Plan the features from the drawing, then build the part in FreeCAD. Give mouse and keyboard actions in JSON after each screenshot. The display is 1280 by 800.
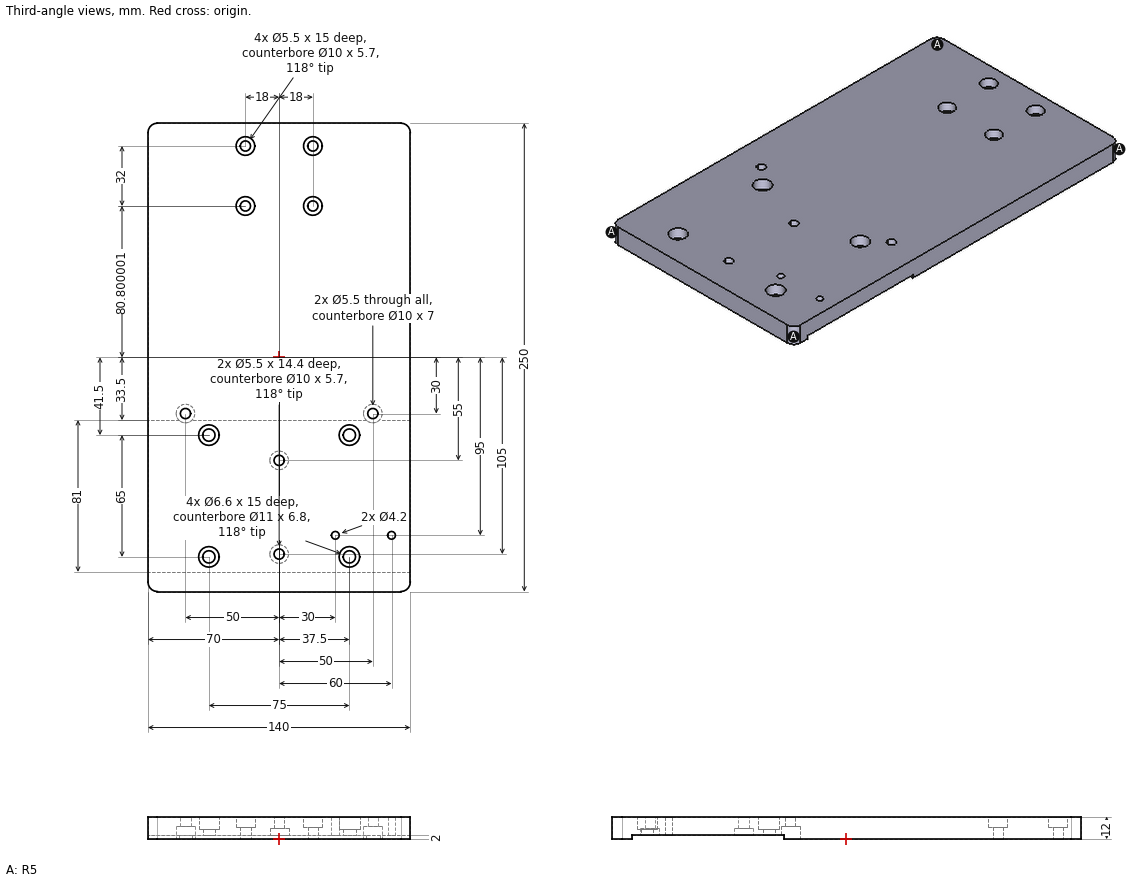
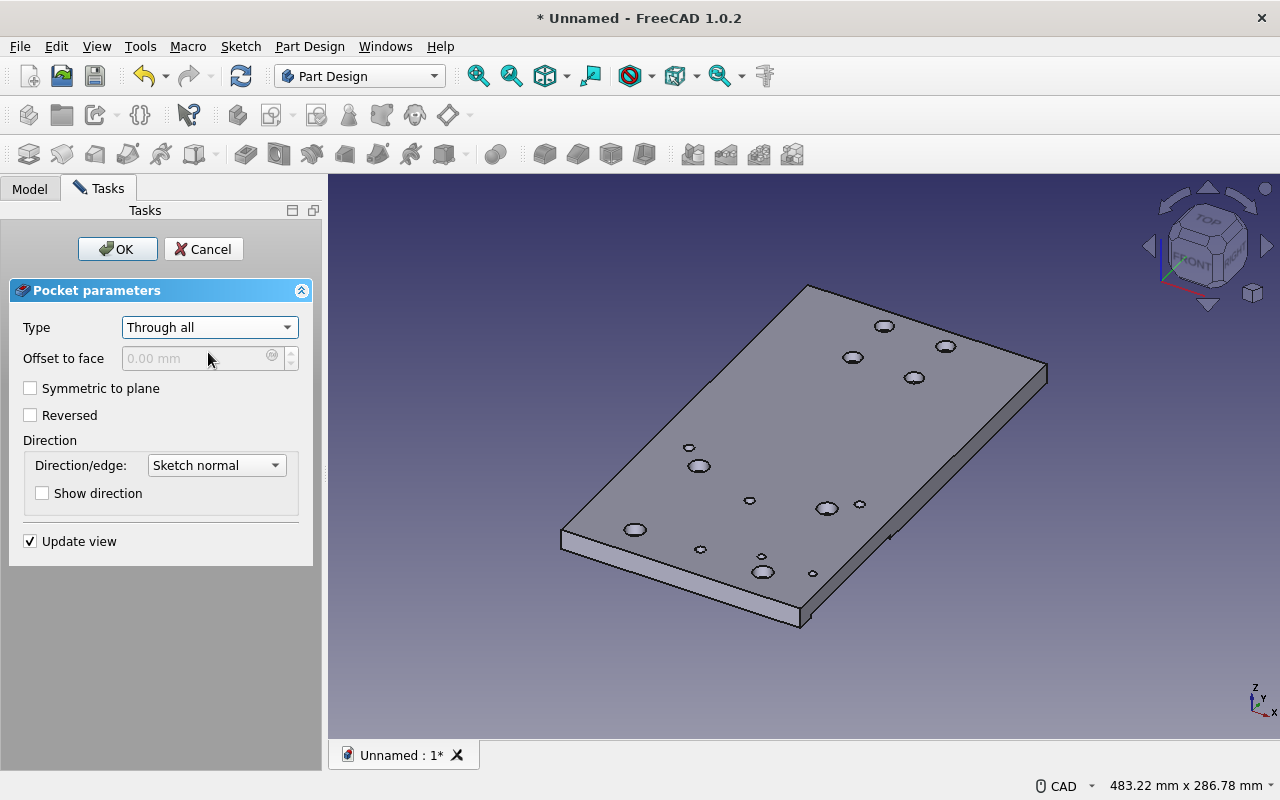
{"action": "left_click", "coordinate": [118, 249]}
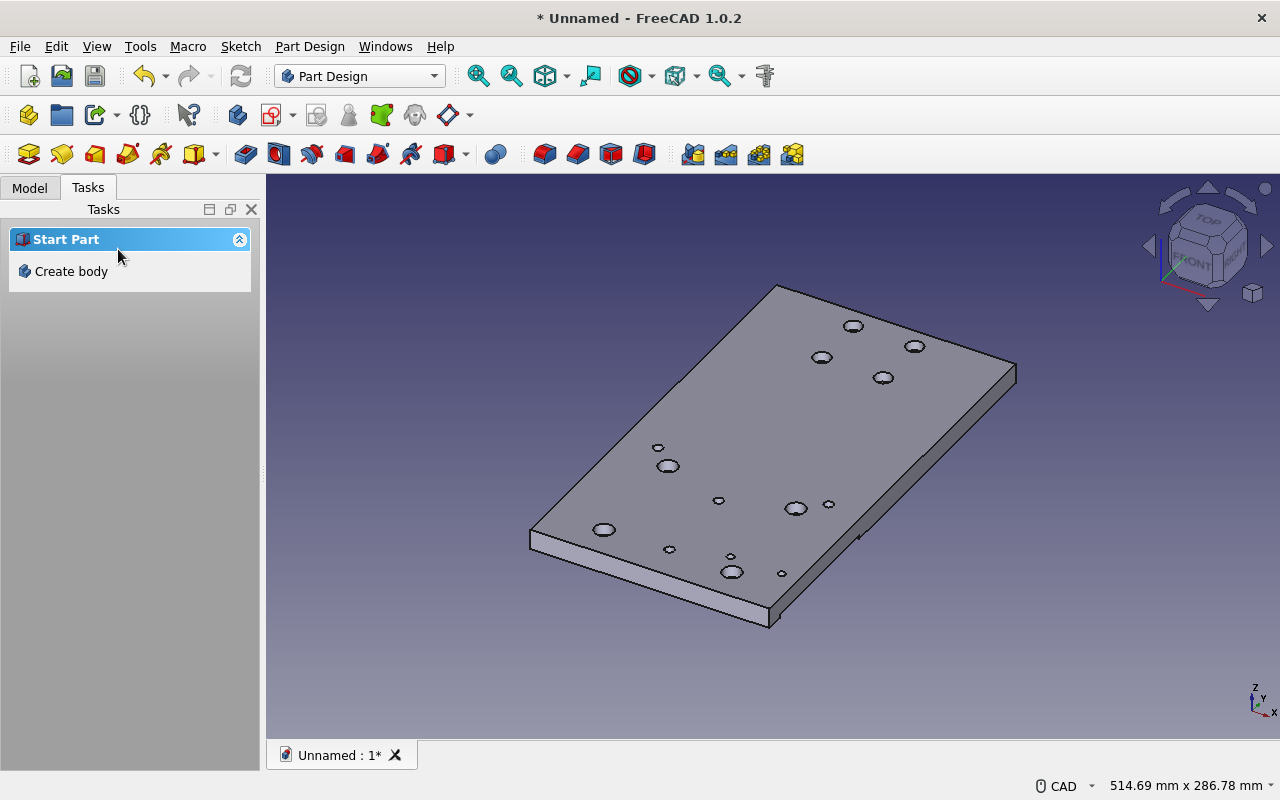
{"action": "left_click", "coordinate": [769, 617]}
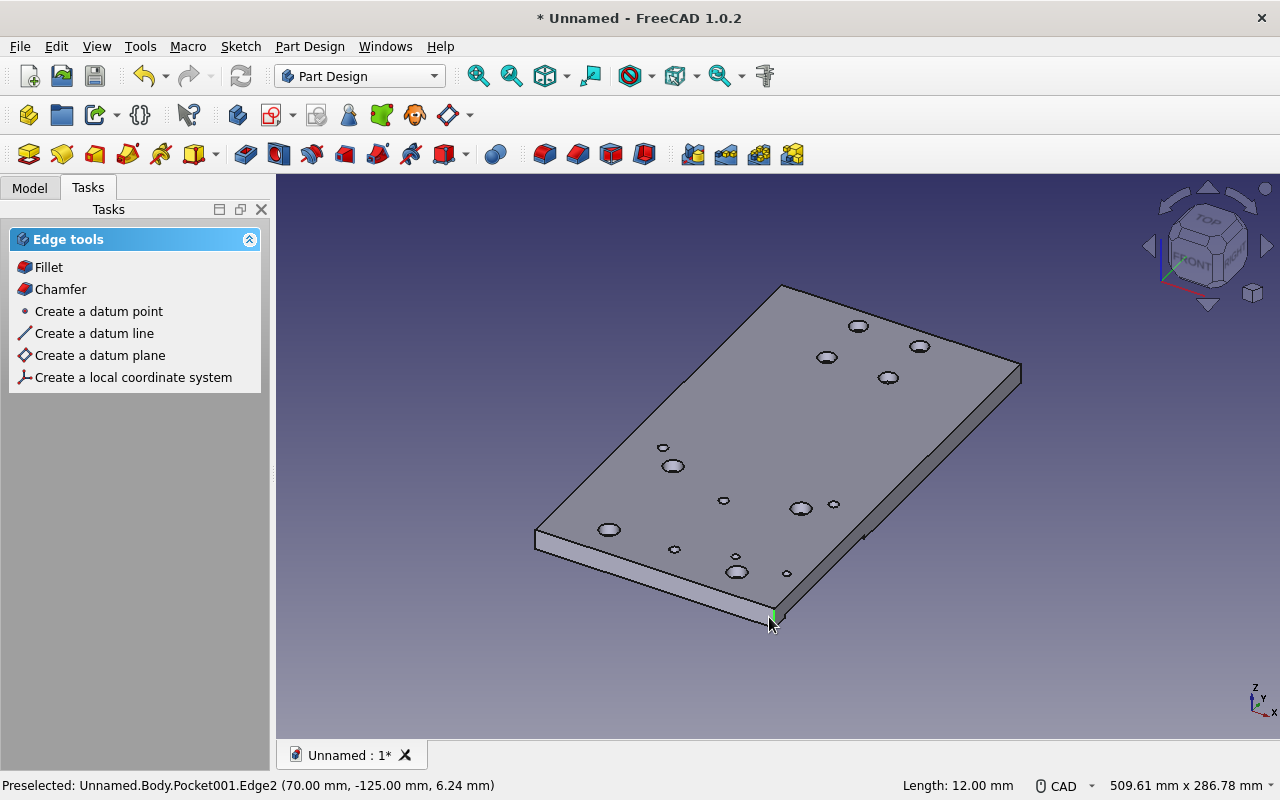
{"action": "key", "text": "0"}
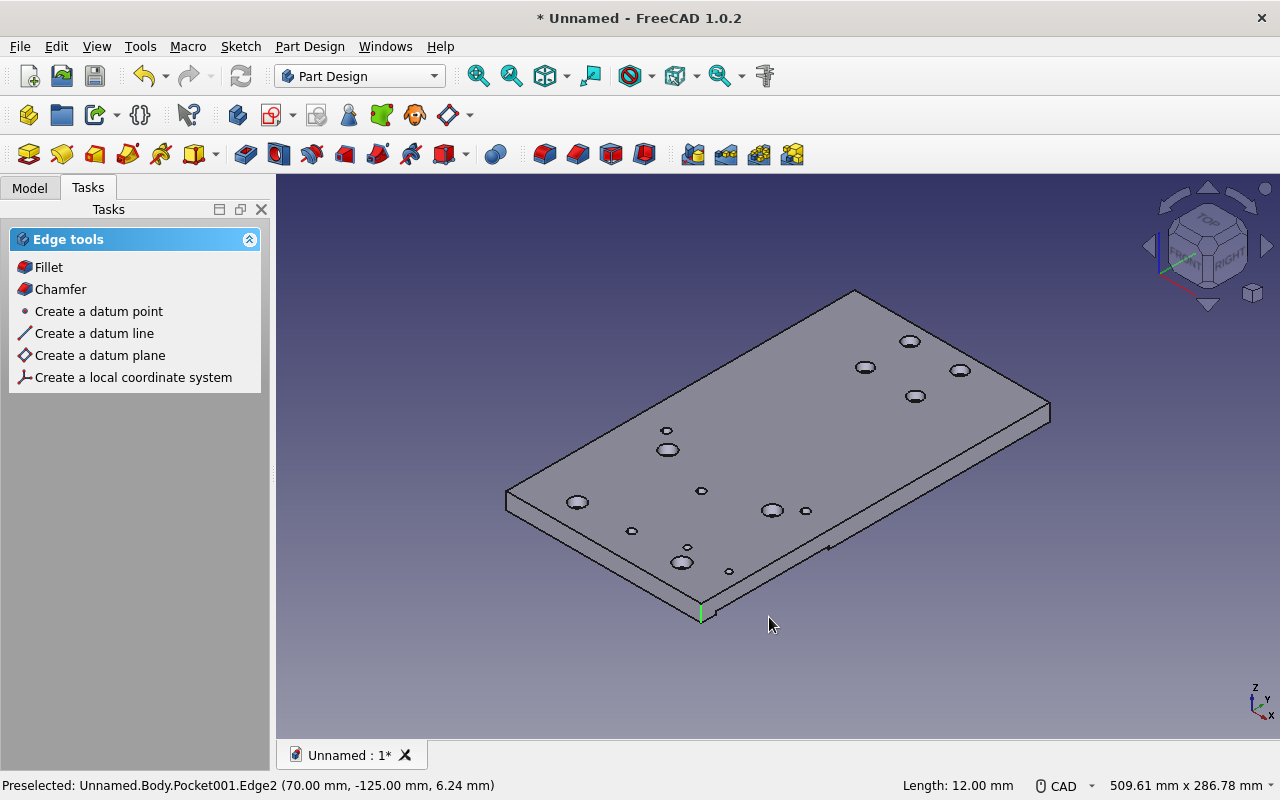
{"action": "key", "text": "2"}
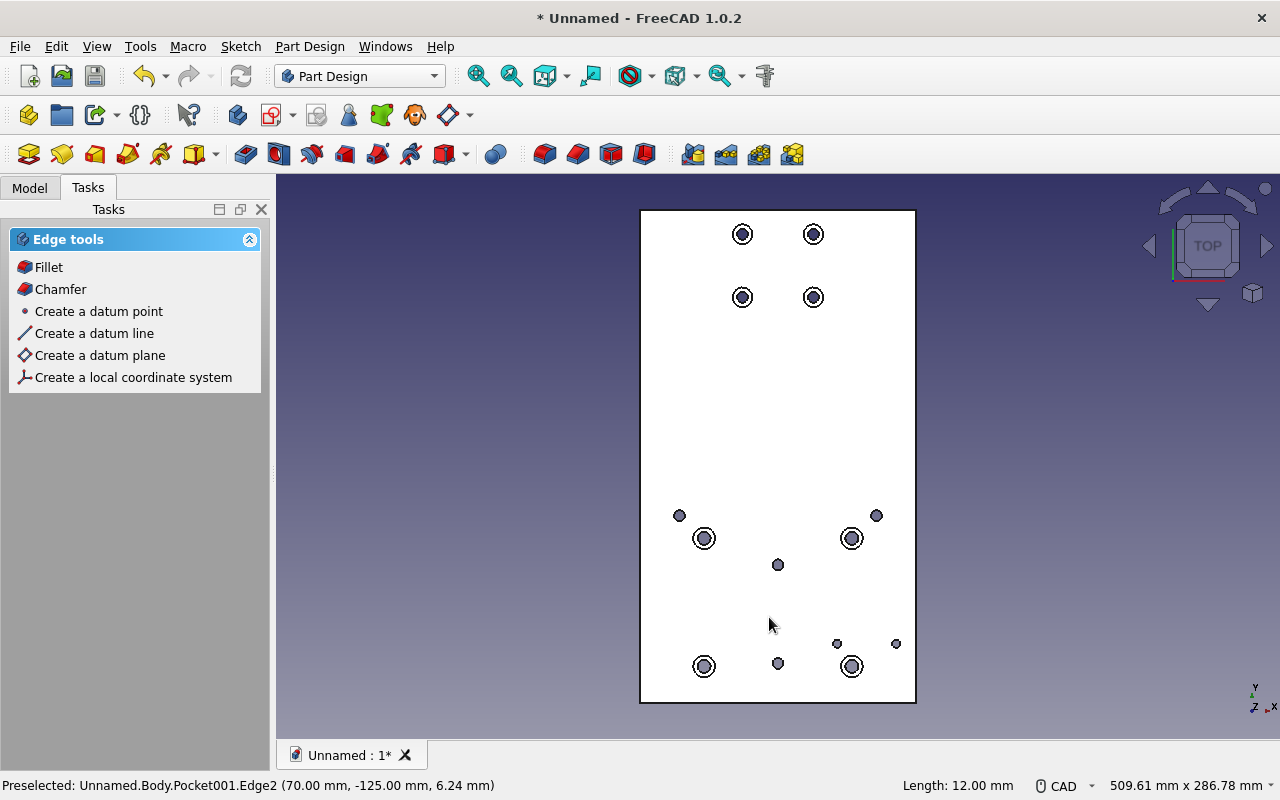
{"action": "key", "text": "1"}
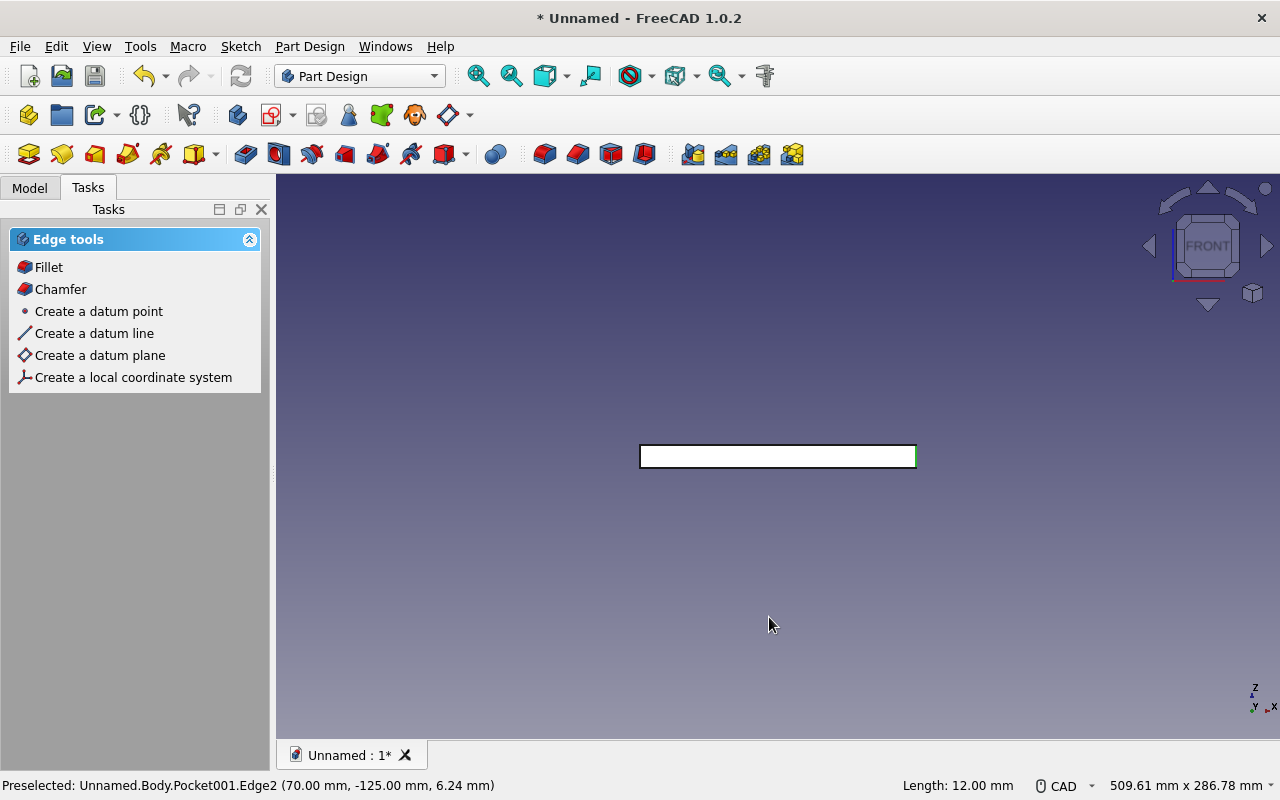
{"action": "left_click", "coordinate": [479, 76]}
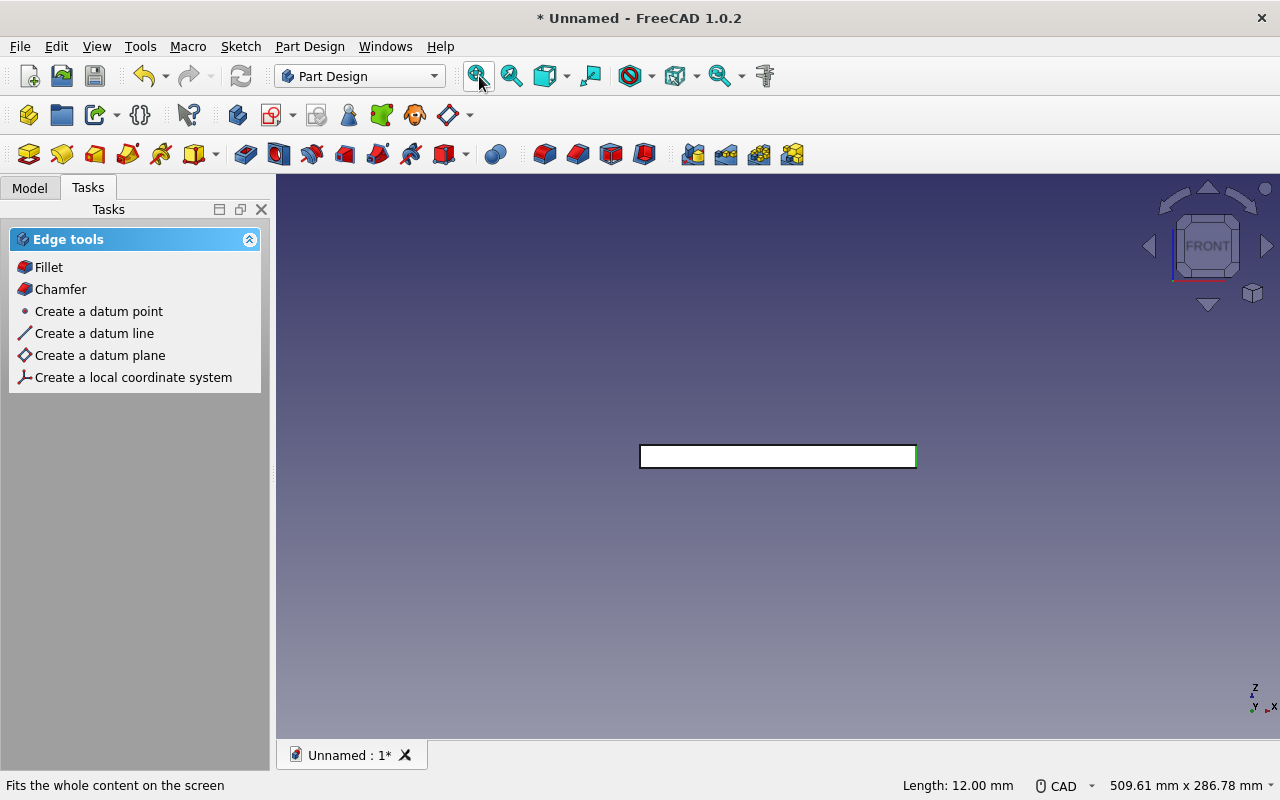
{"action": "left_click", "coordinate": [640, 456], "text": "ctrl"}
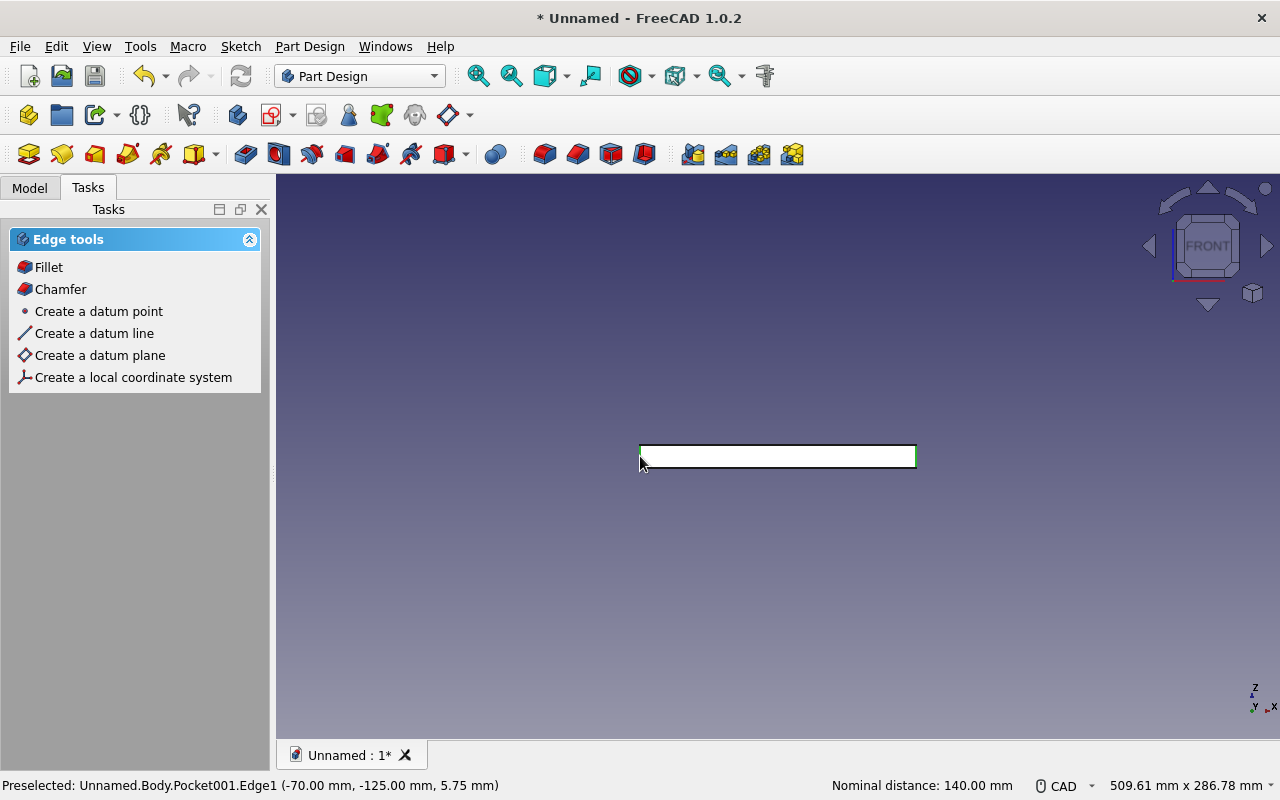
{"action": "key", "text": "3"}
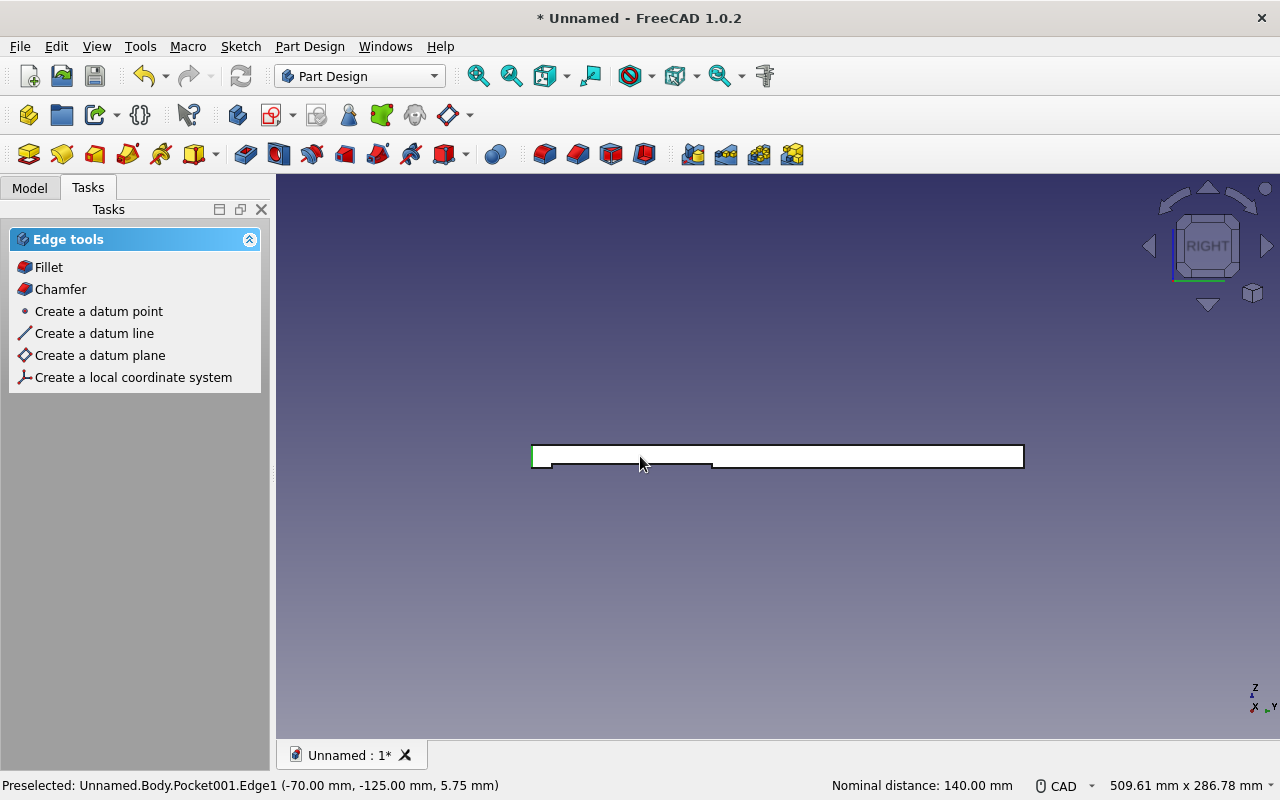
{"action": "left_click", "coordinate": [1024, 455], "text": "ctrl"}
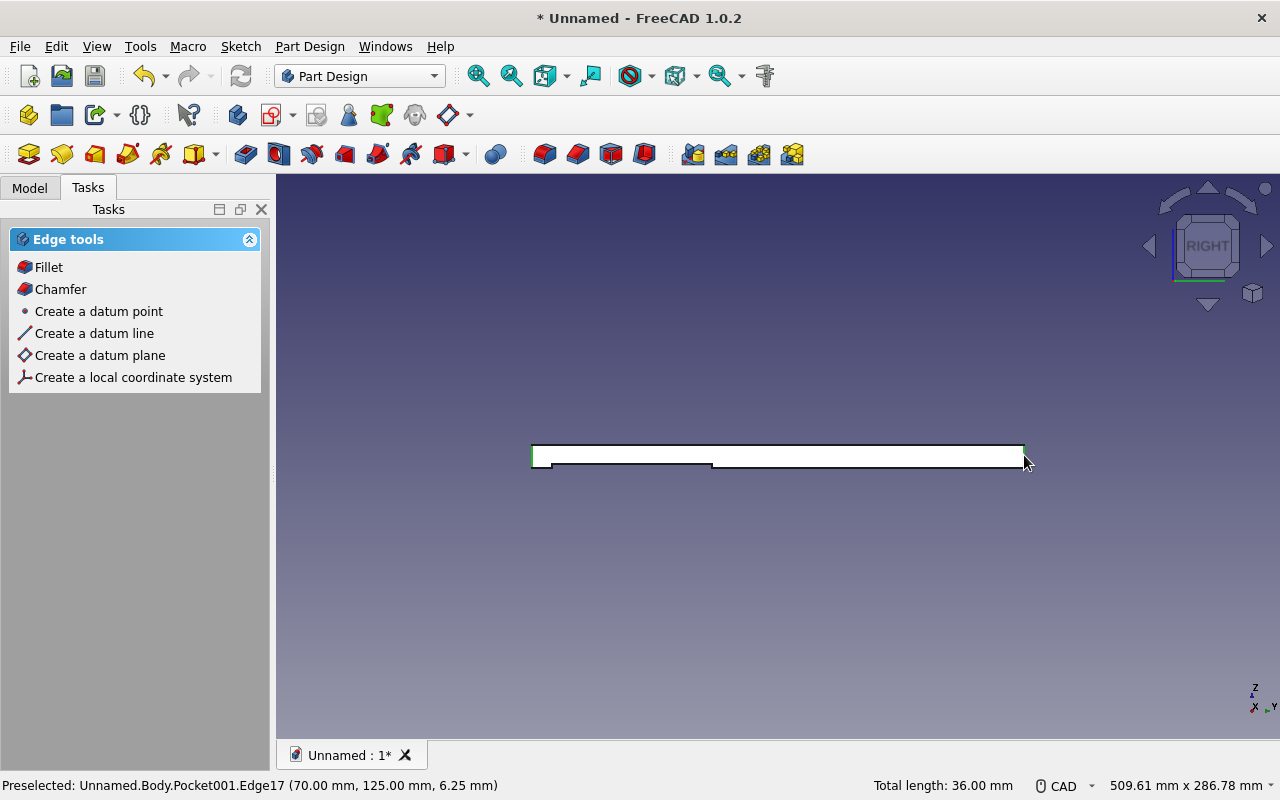
{"action": "key", "text": "5"}